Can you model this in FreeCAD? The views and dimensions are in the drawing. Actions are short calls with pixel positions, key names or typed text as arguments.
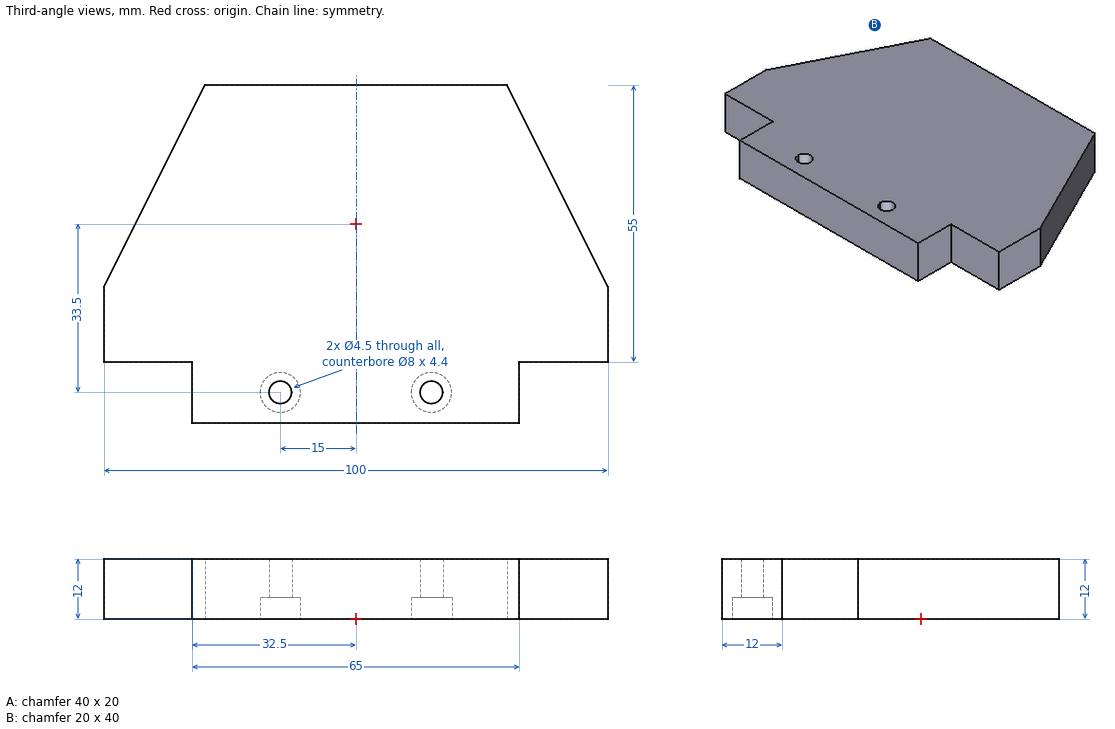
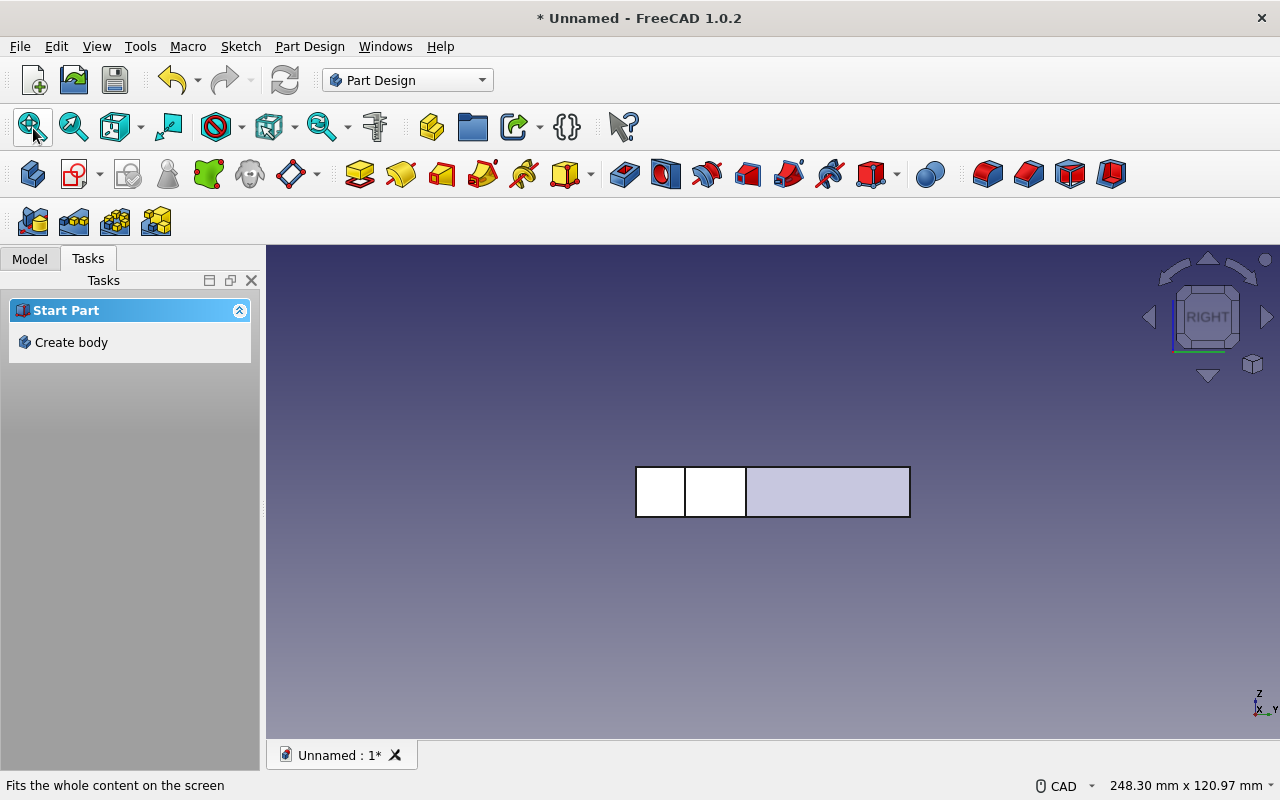
key(5)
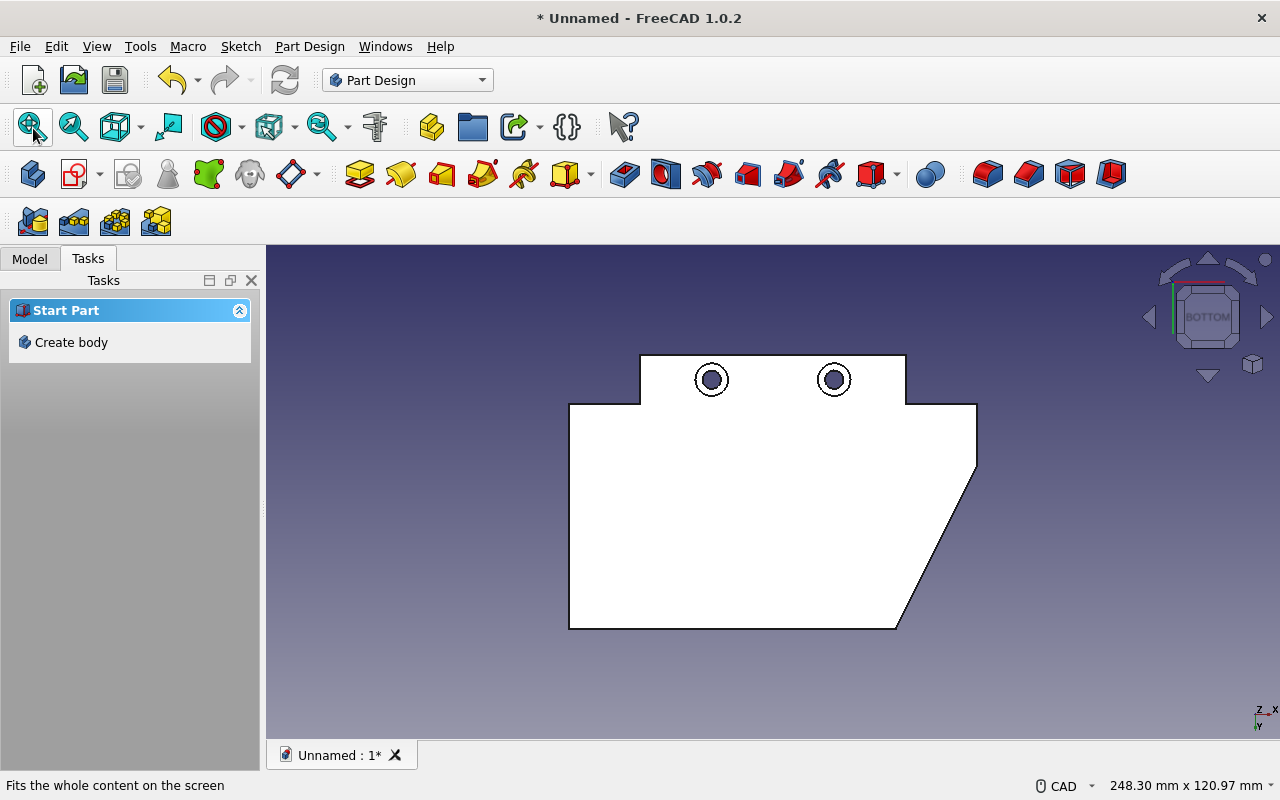
key(4)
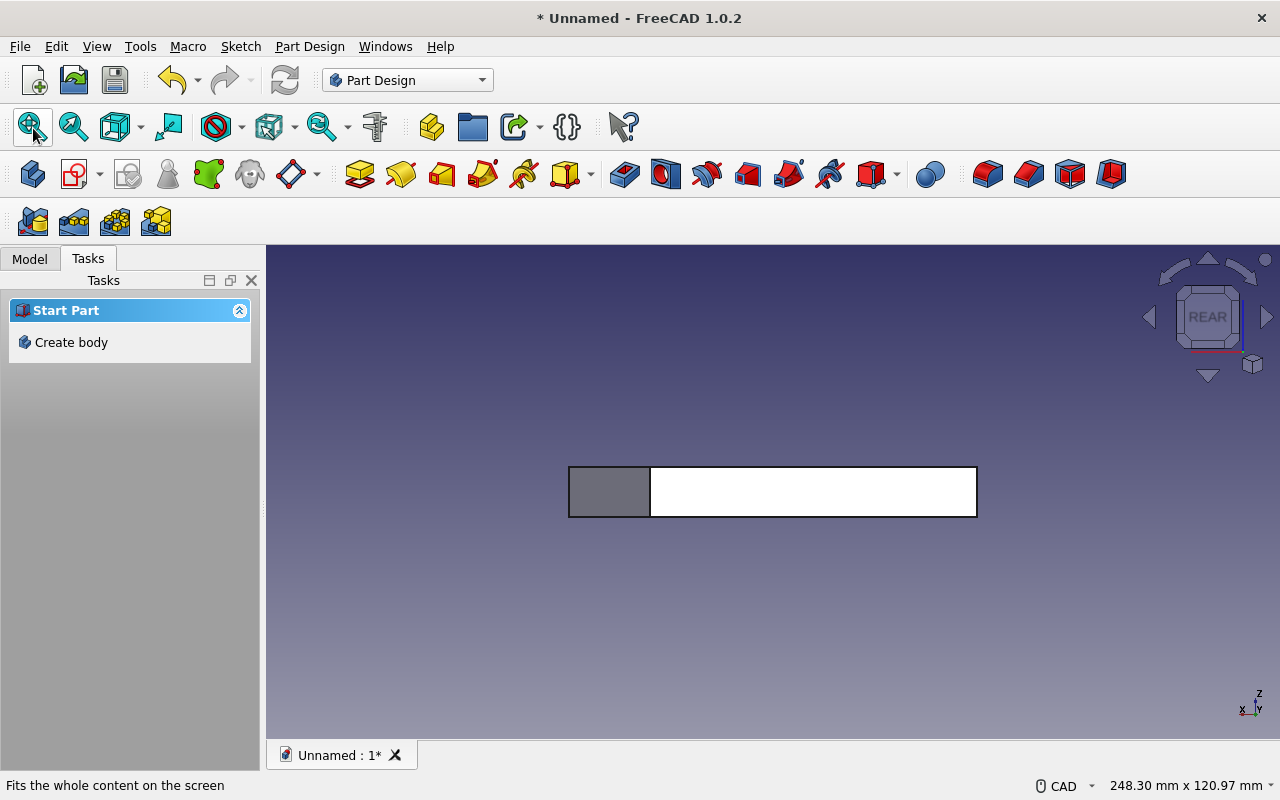
click(33, 128)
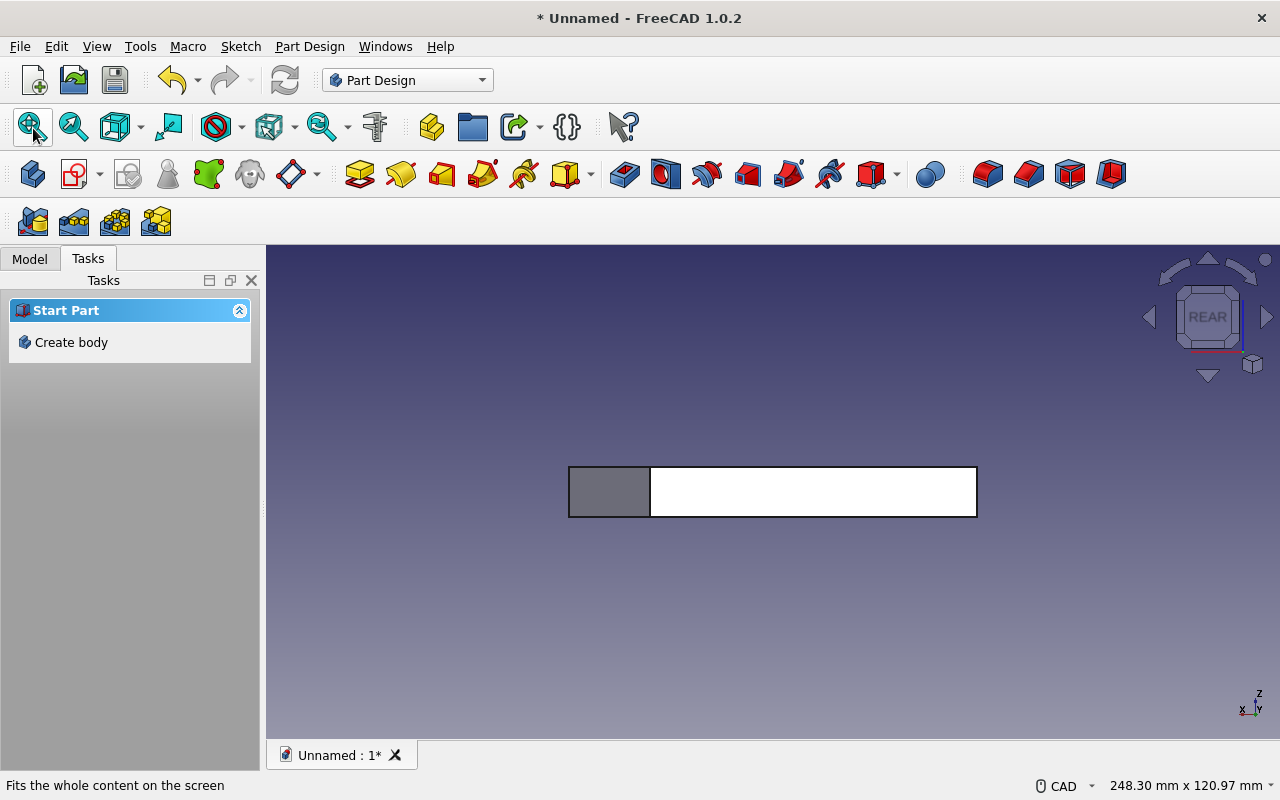
click(977, 491)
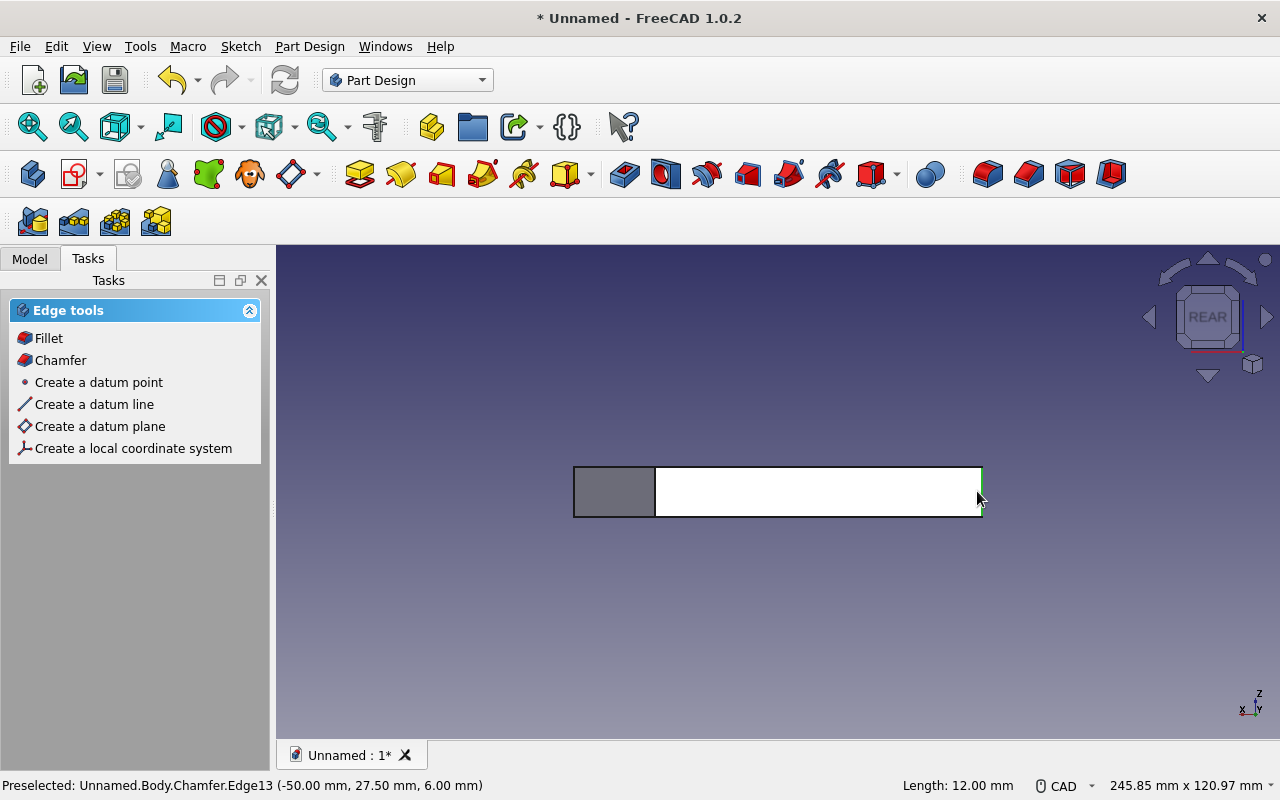
click(1029, 174)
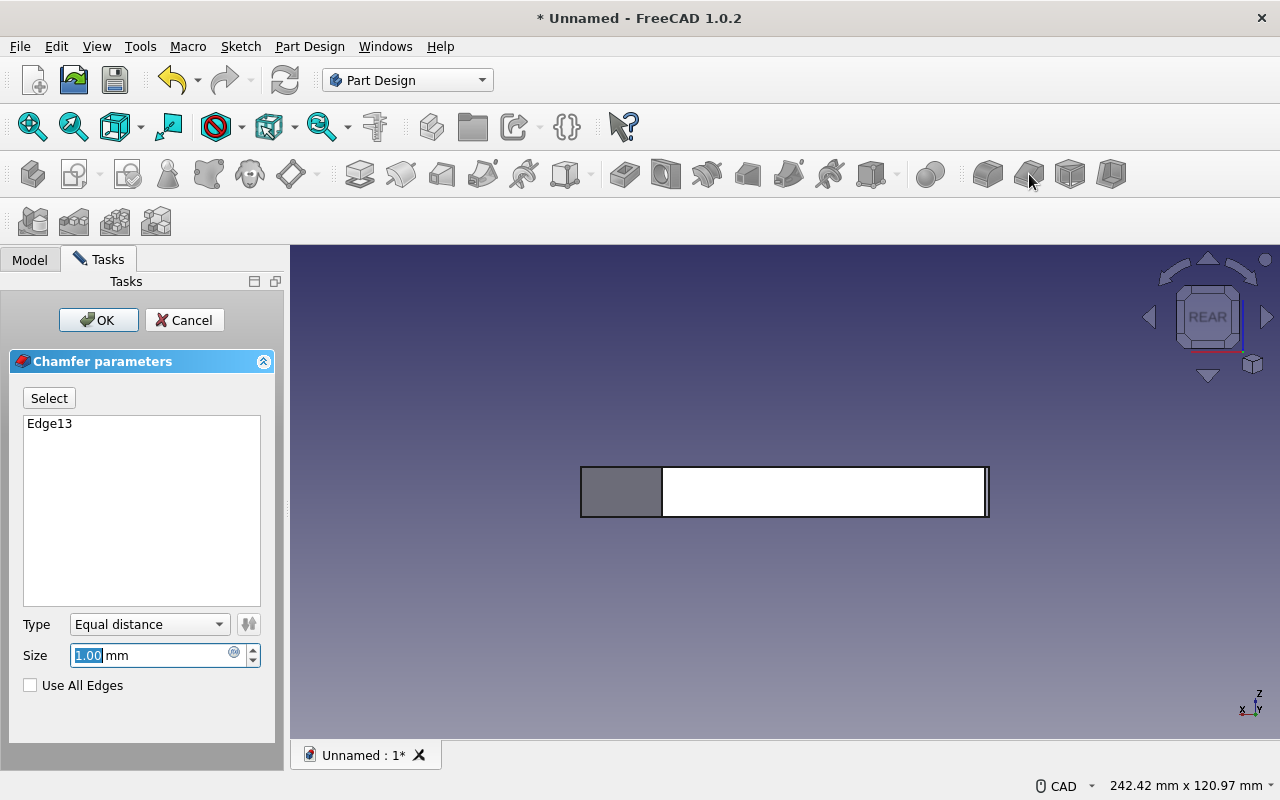
text(20)
key(Tab)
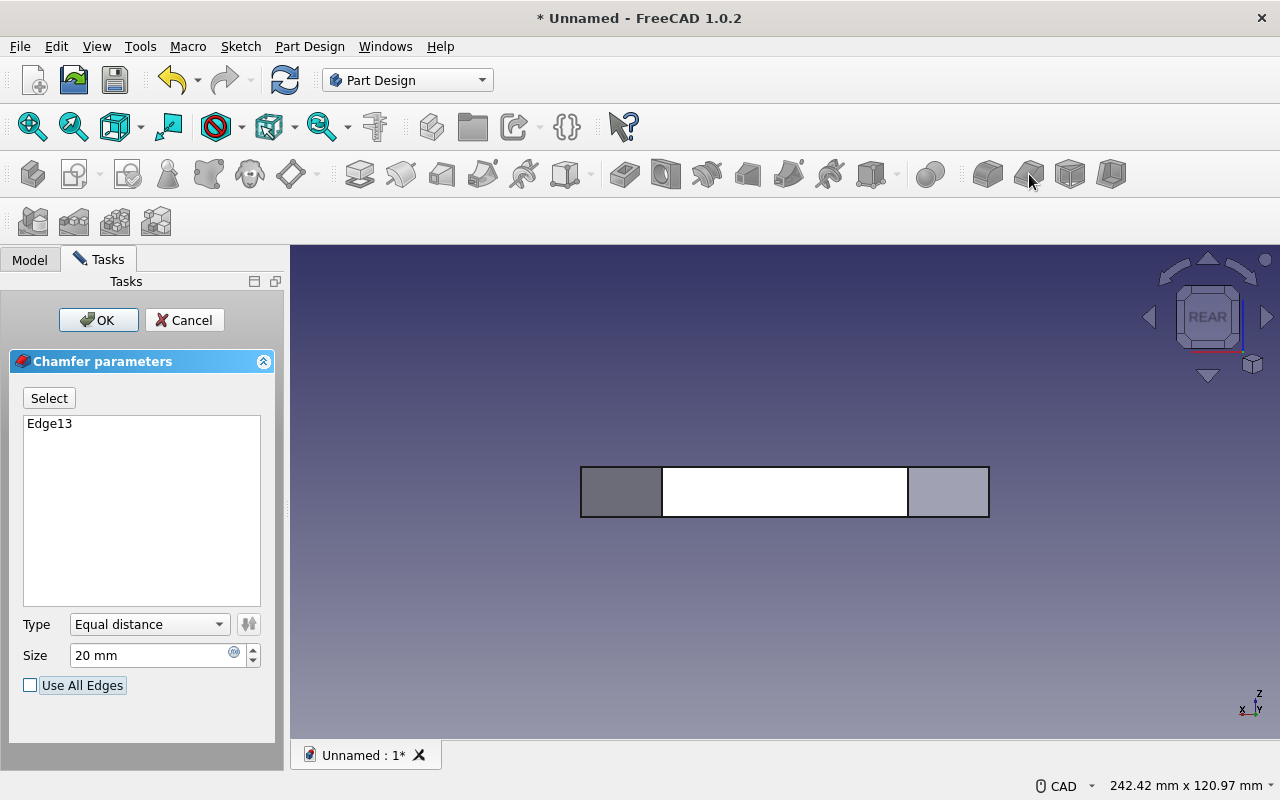
click(150, 624)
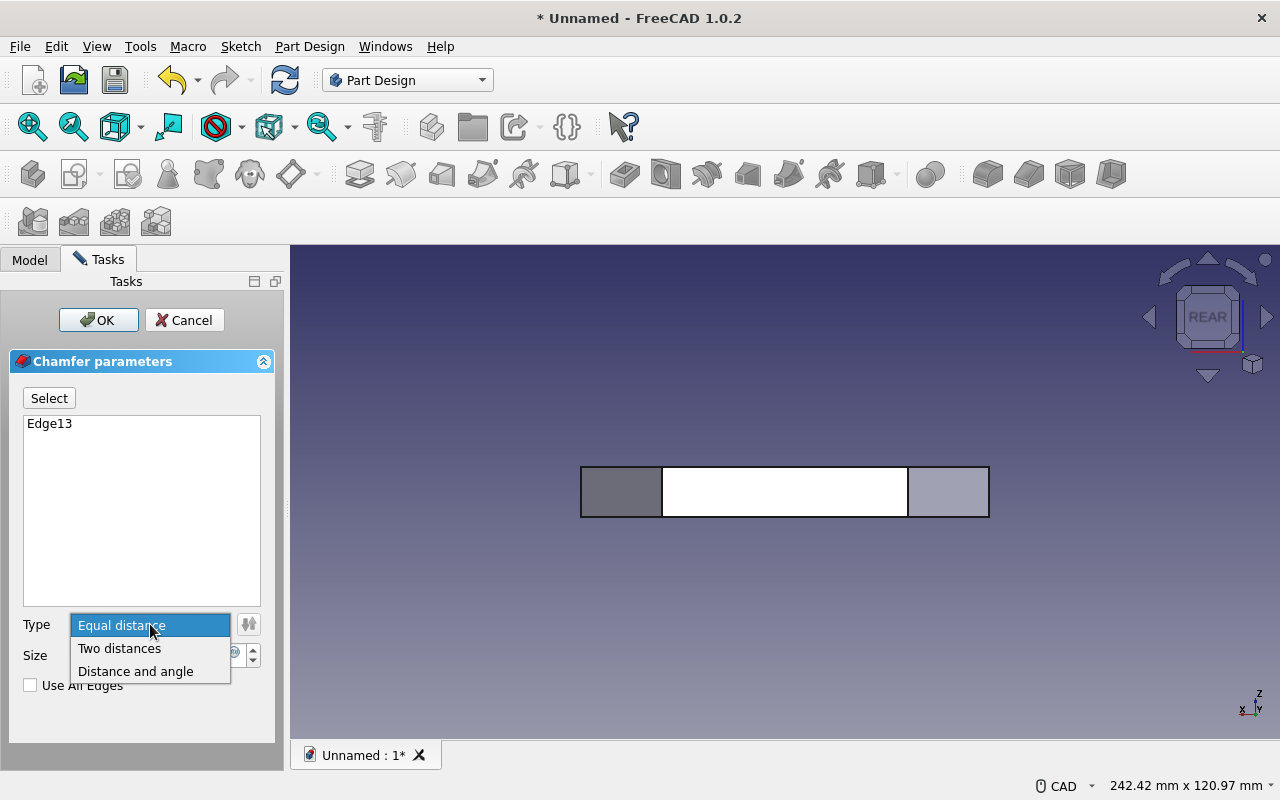
click(148, 648)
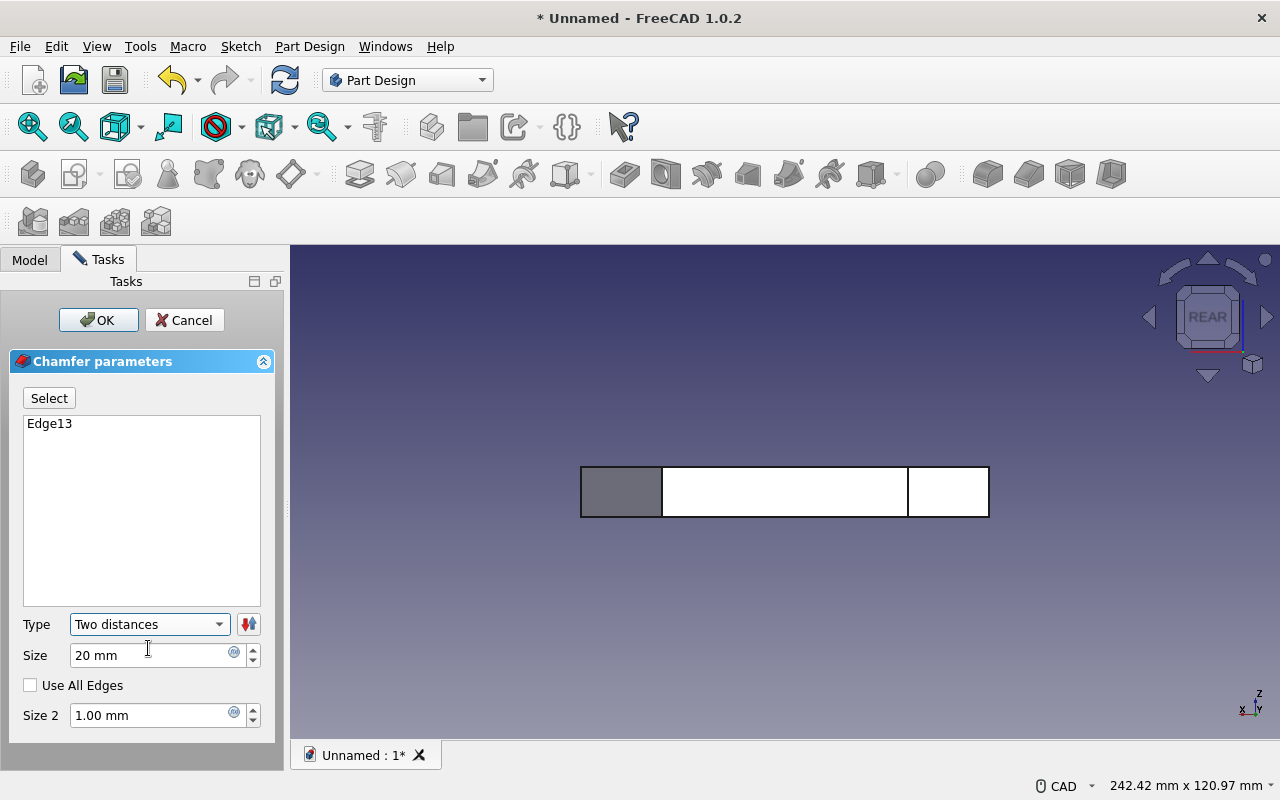
triple_click(158, 716)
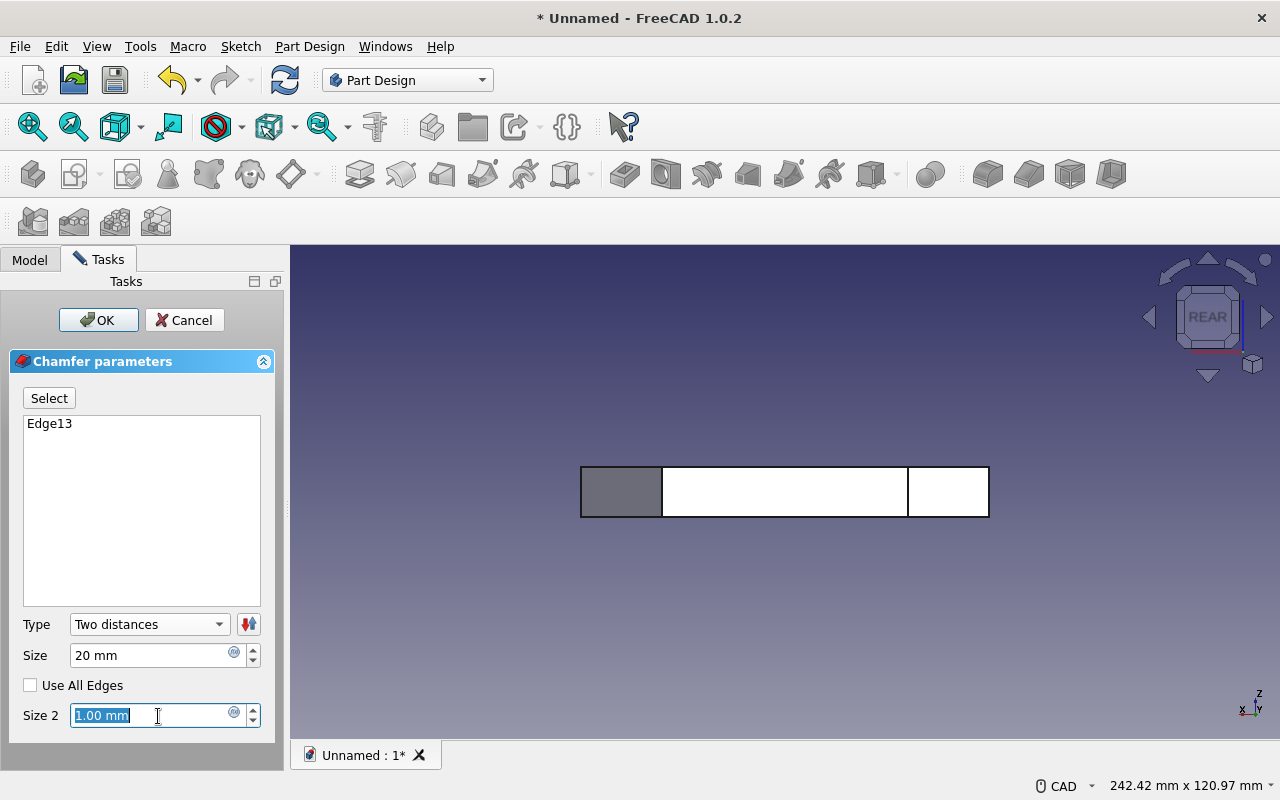
text(40)
key(Tab)